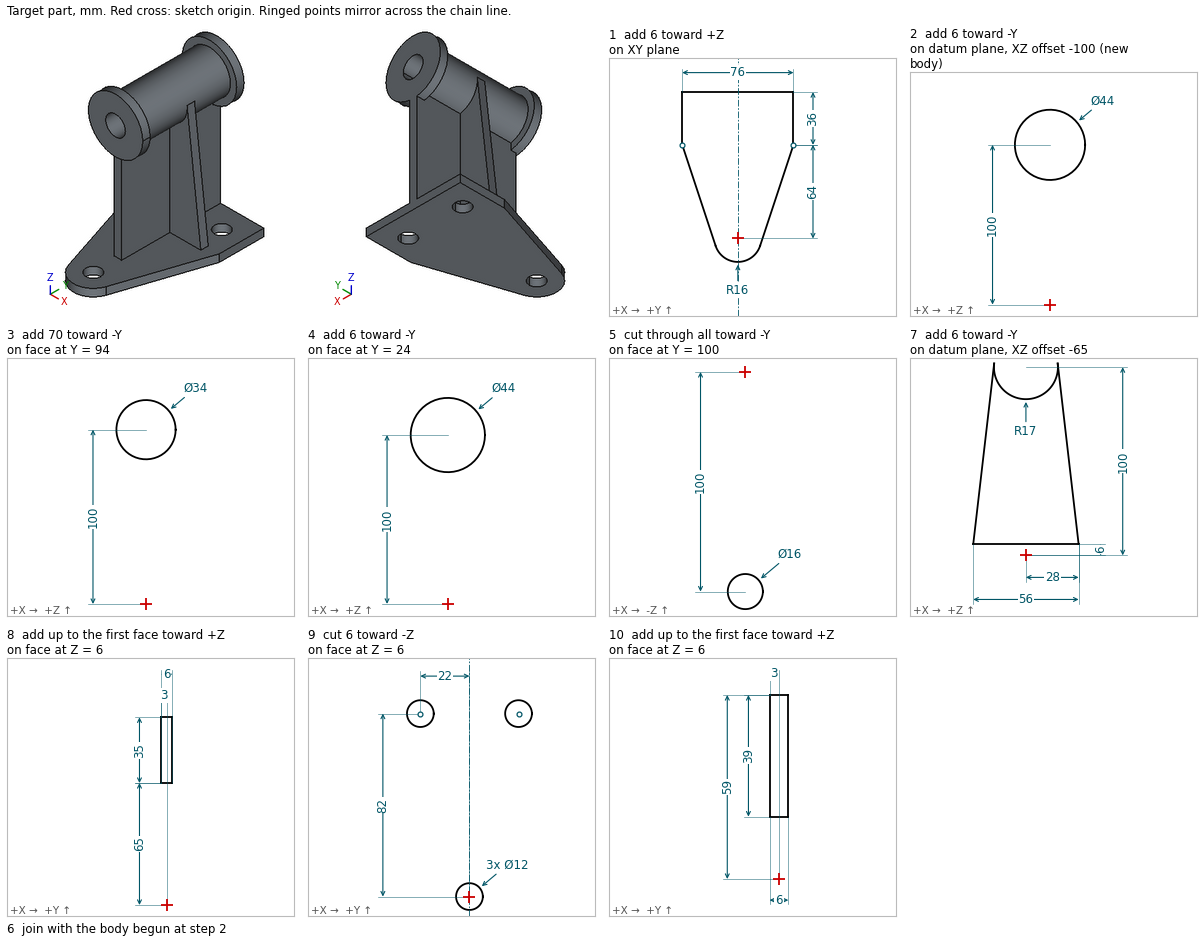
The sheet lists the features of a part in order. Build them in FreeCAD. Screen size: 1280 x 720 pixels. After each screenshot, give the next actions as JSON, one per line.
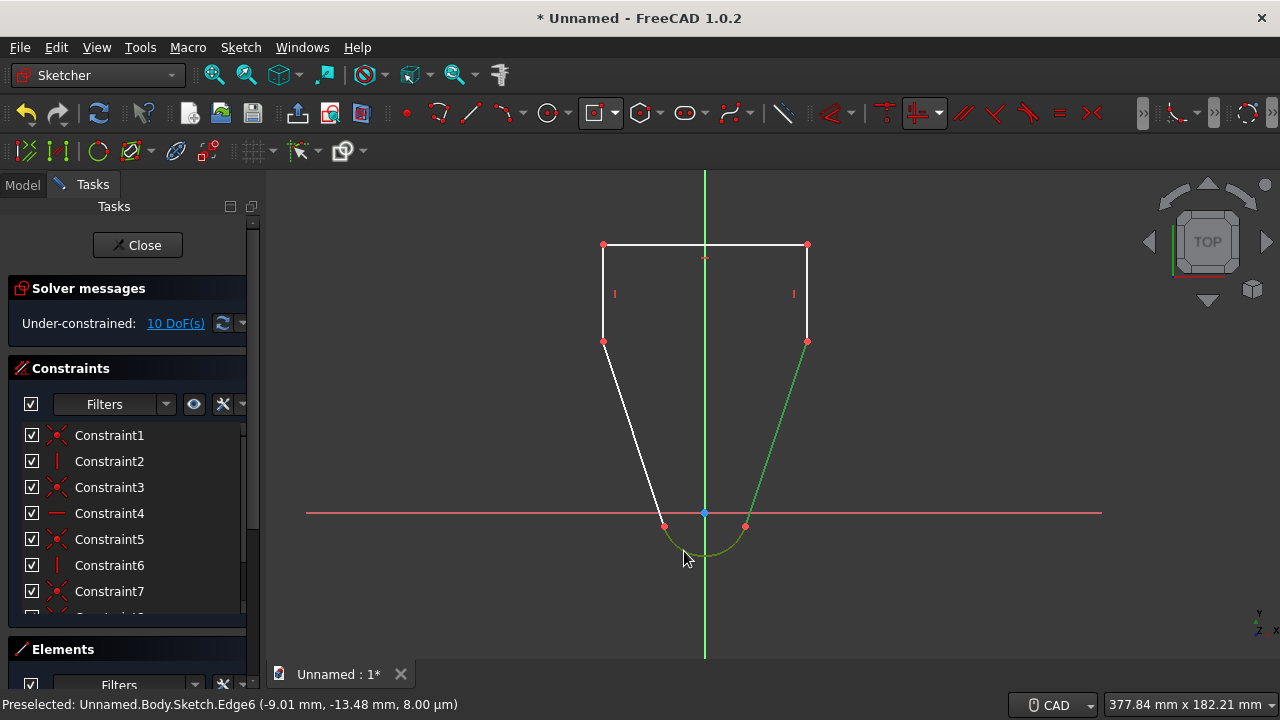
{"action": "key", "text": "t"}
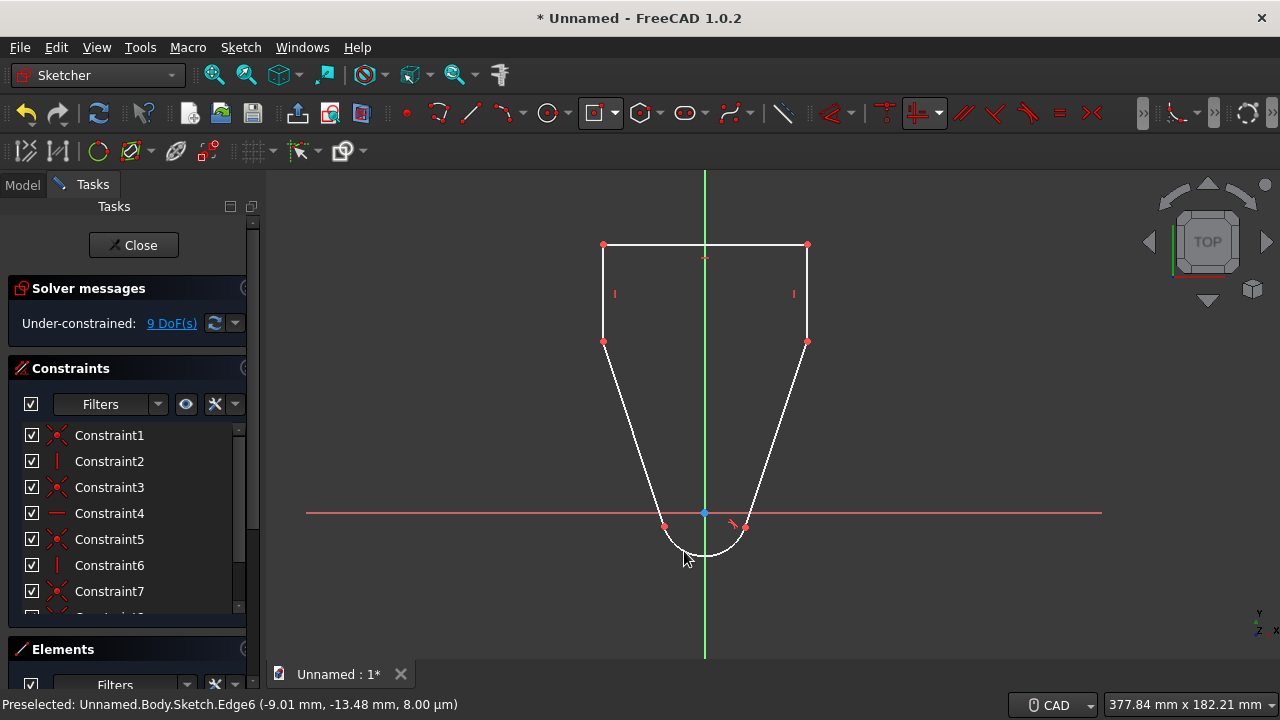
{"action": "left_click", "coordinate": [621, 397]}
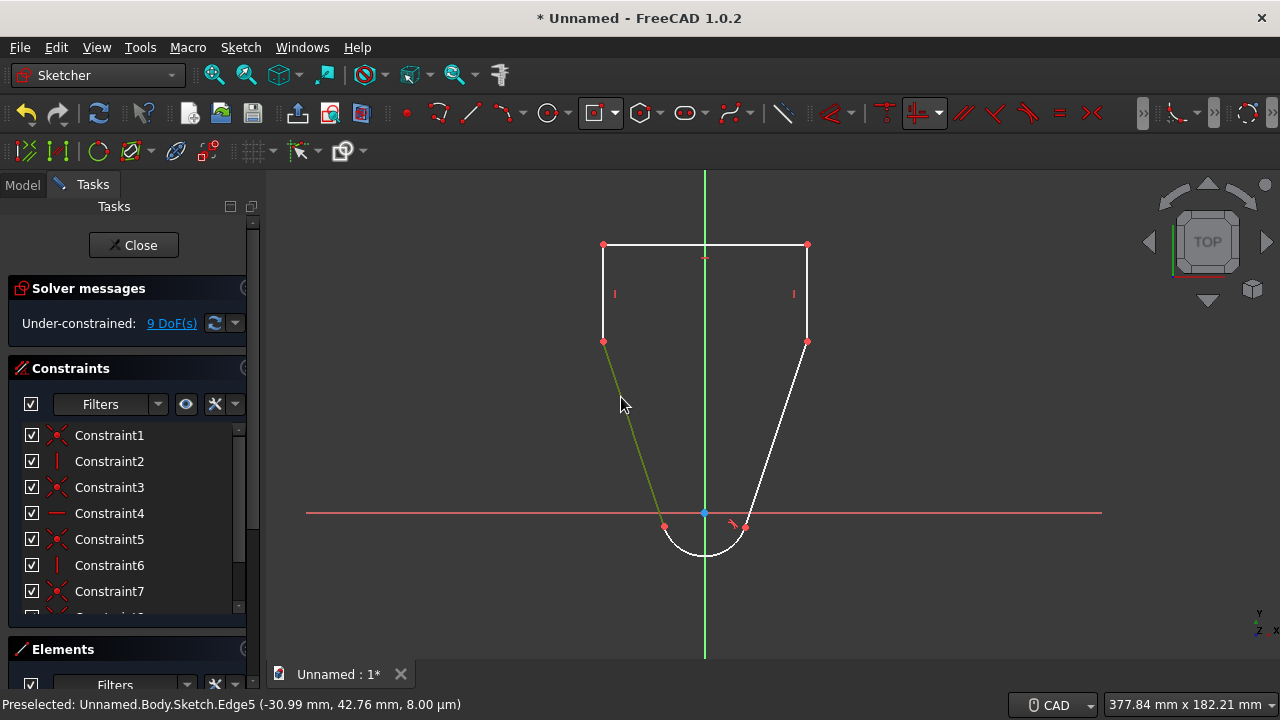
{"action": "left_click", "coordinate": [684, 551]}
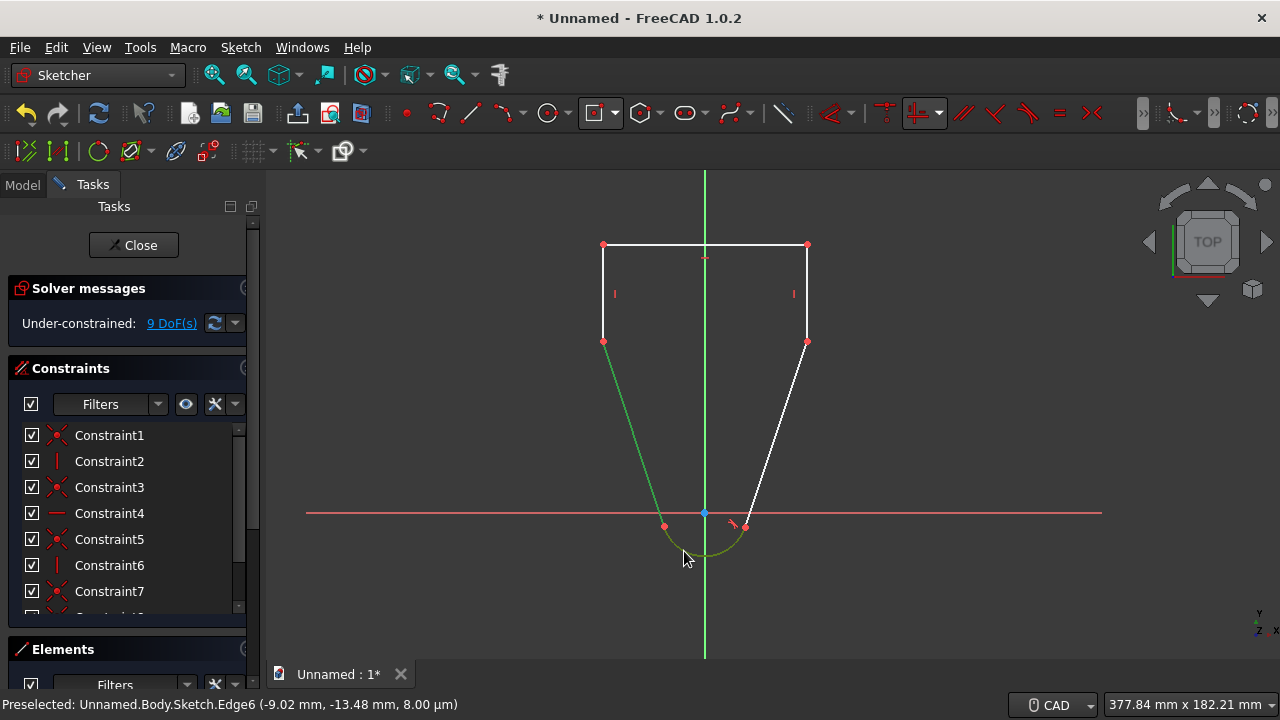
{"action": "key", "text": "t"}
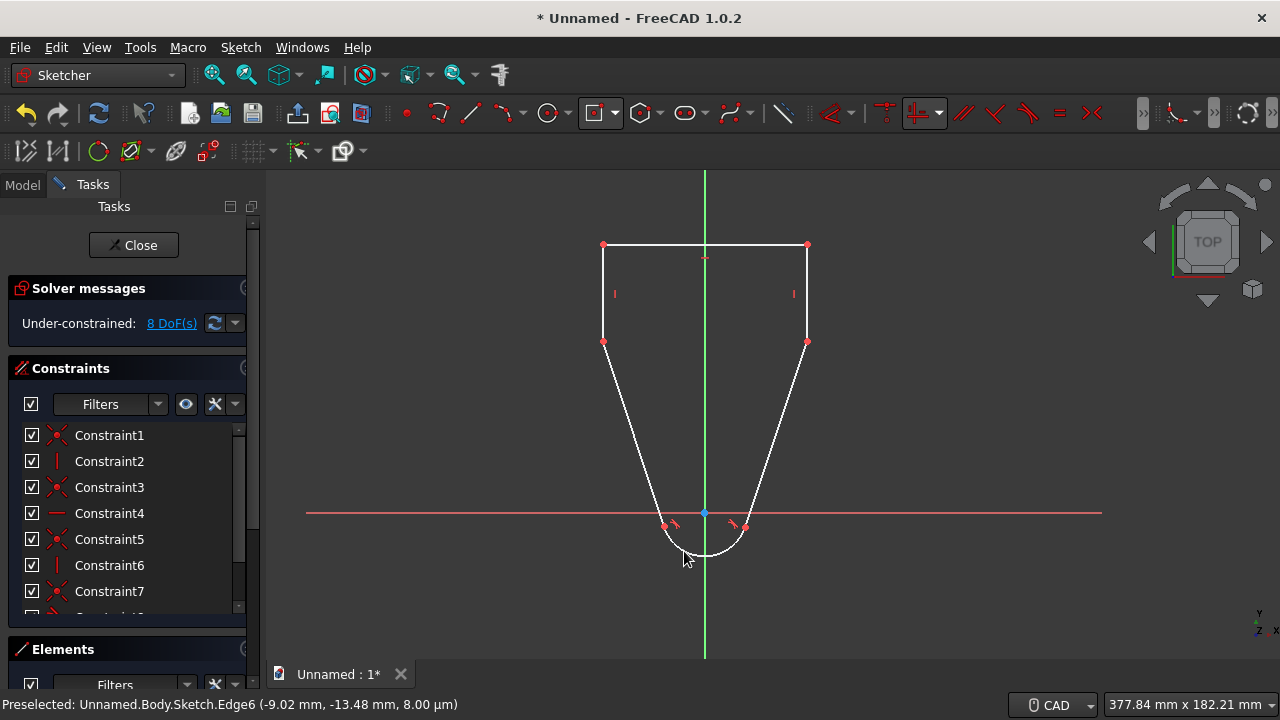
{"action": "left_click_drag", "start_coordinate": [695, 503], "coordinate": [715, 524]}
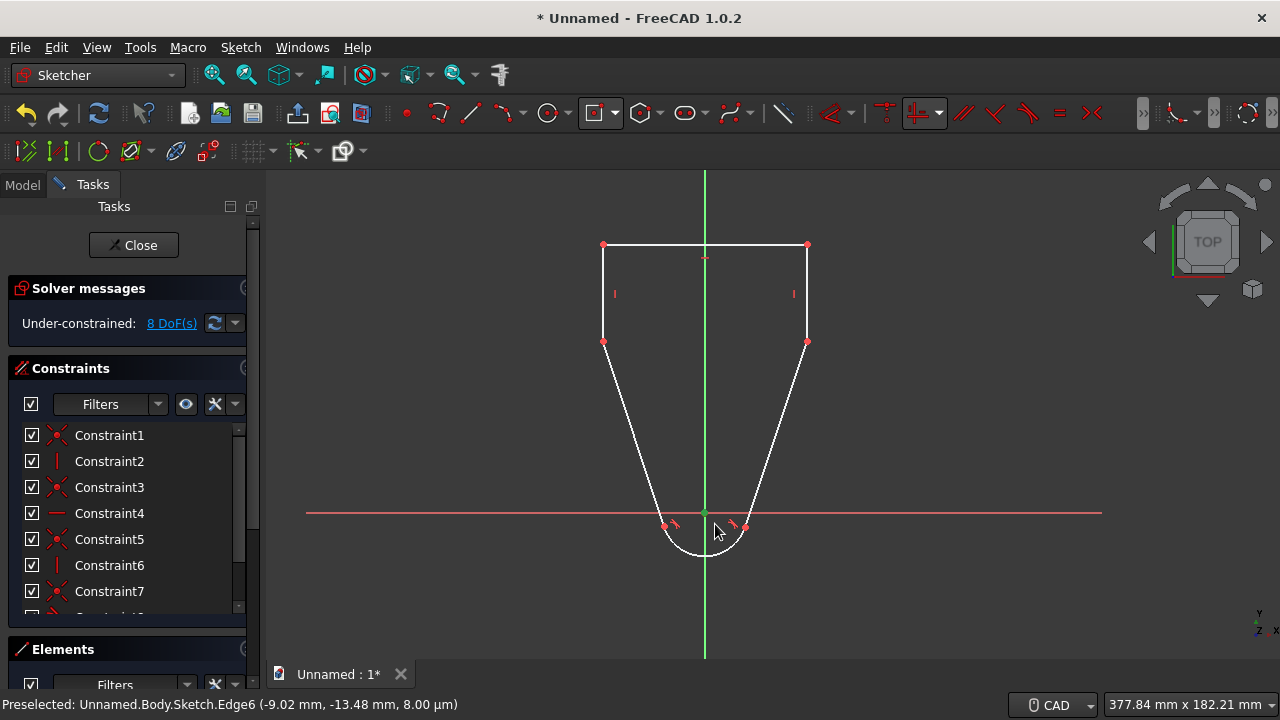
{"action": "key", "text": "c"}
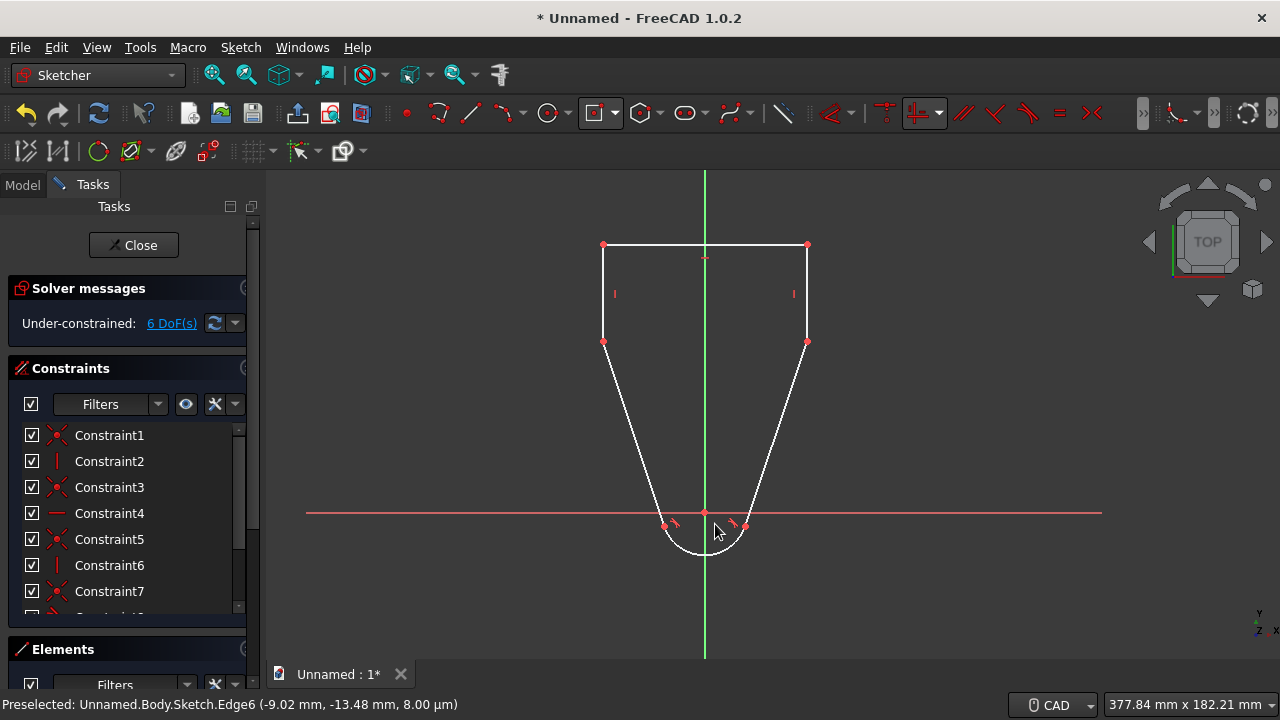
{"action": "left_click", "coordinate": [807, 342]}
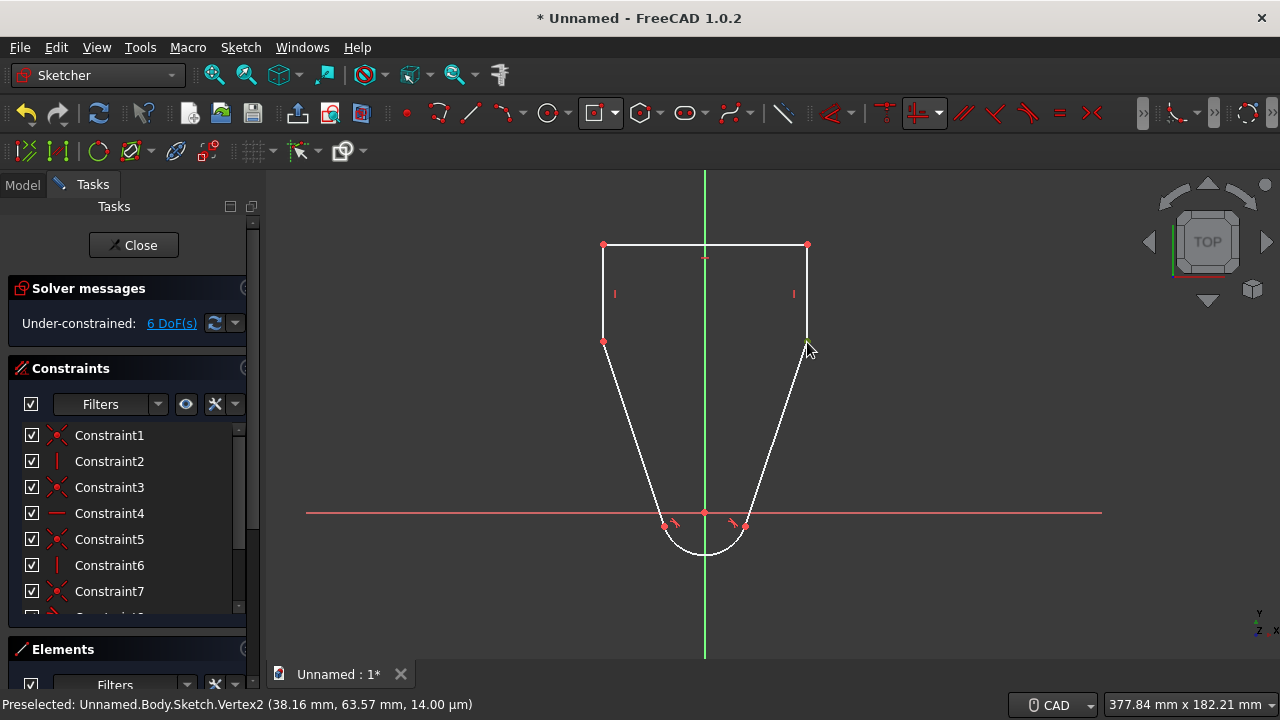
{"action": "left_click", "coordinate": [603, 342]}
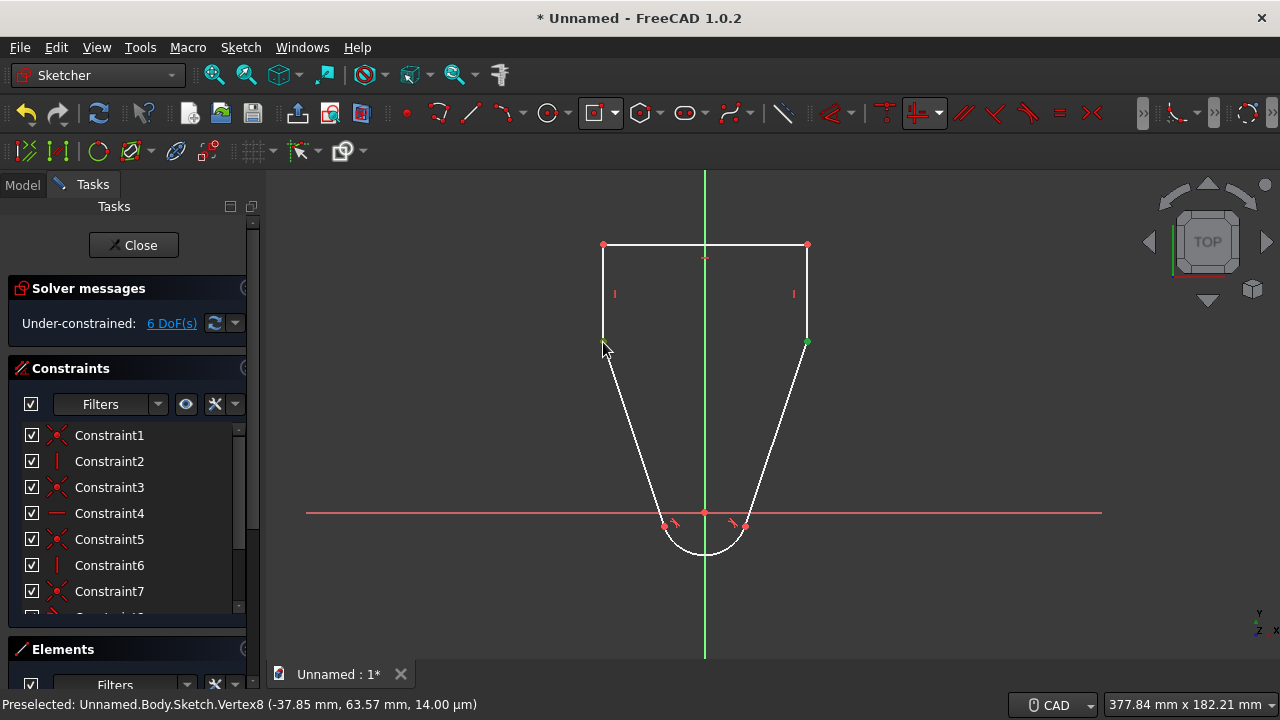
{"action": "left_click", "coordinate": [705, 600]}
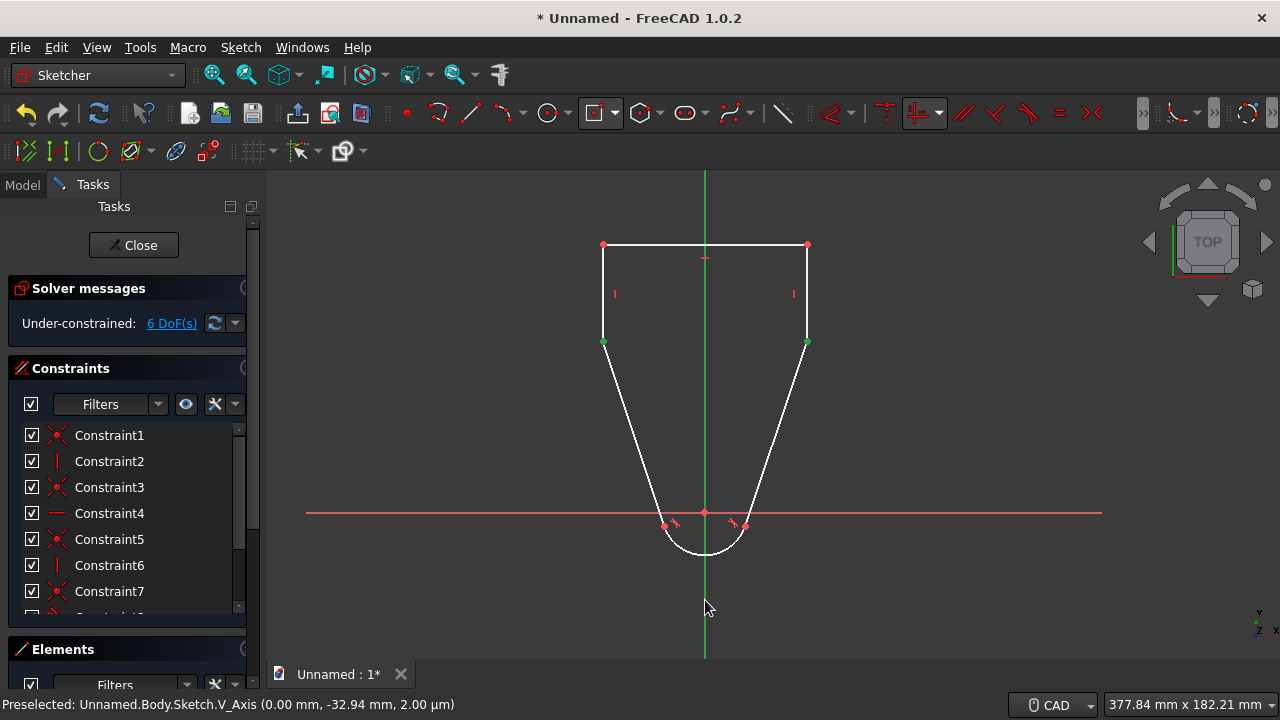
{"action": "key", "text": "s"}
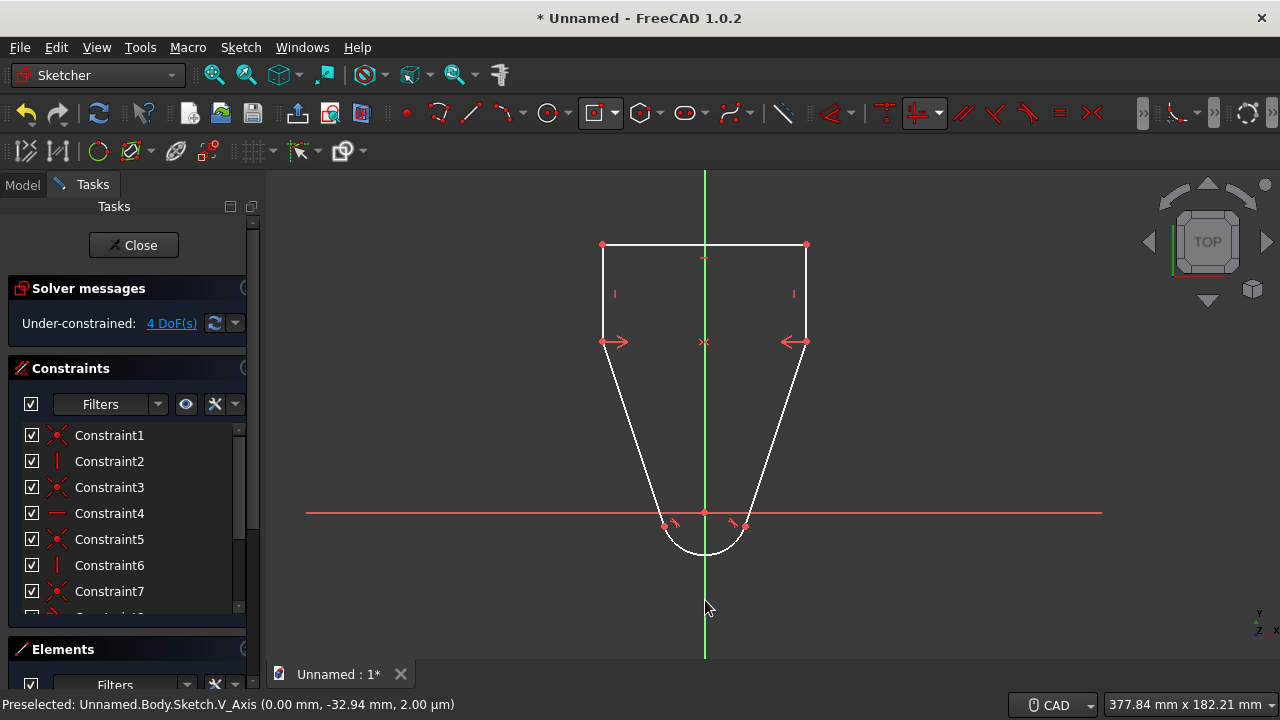
{"action": "key", "text": "d"}